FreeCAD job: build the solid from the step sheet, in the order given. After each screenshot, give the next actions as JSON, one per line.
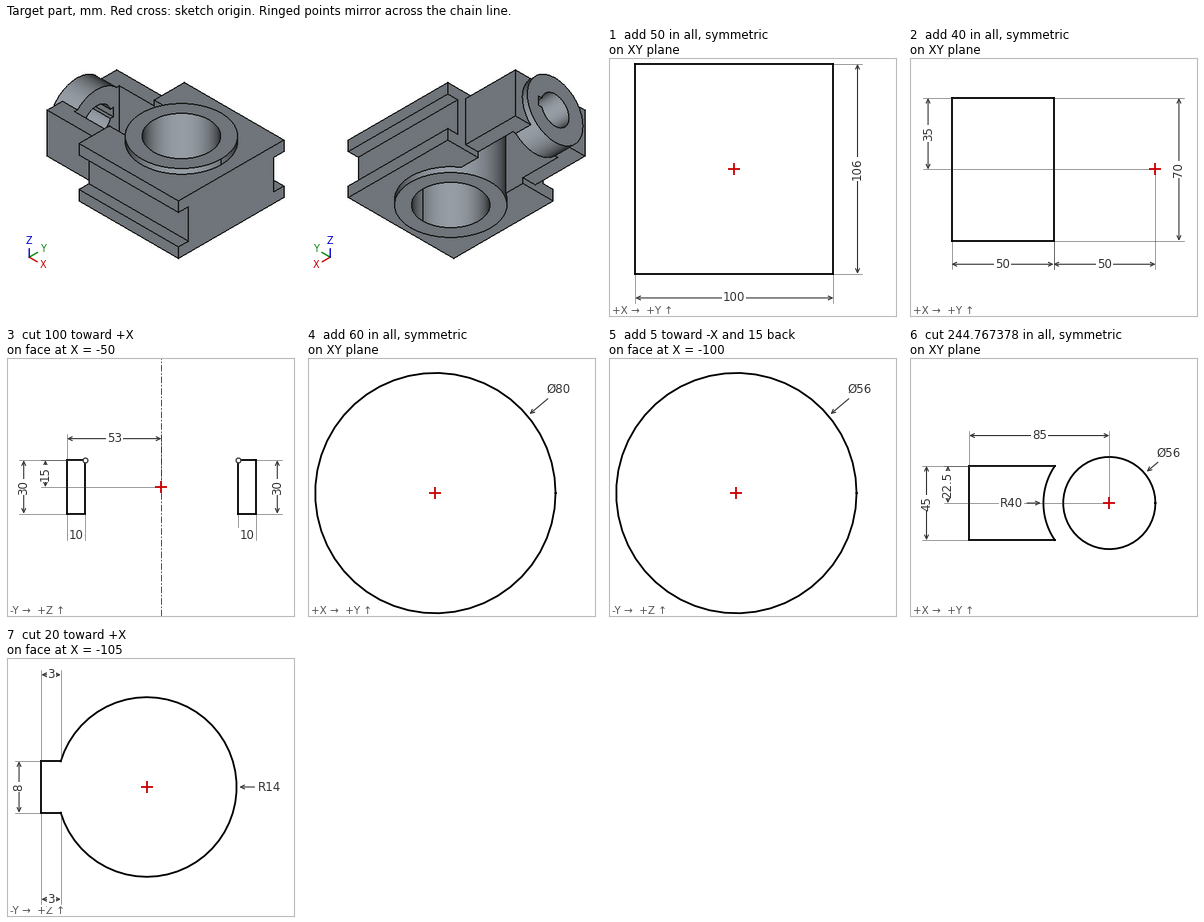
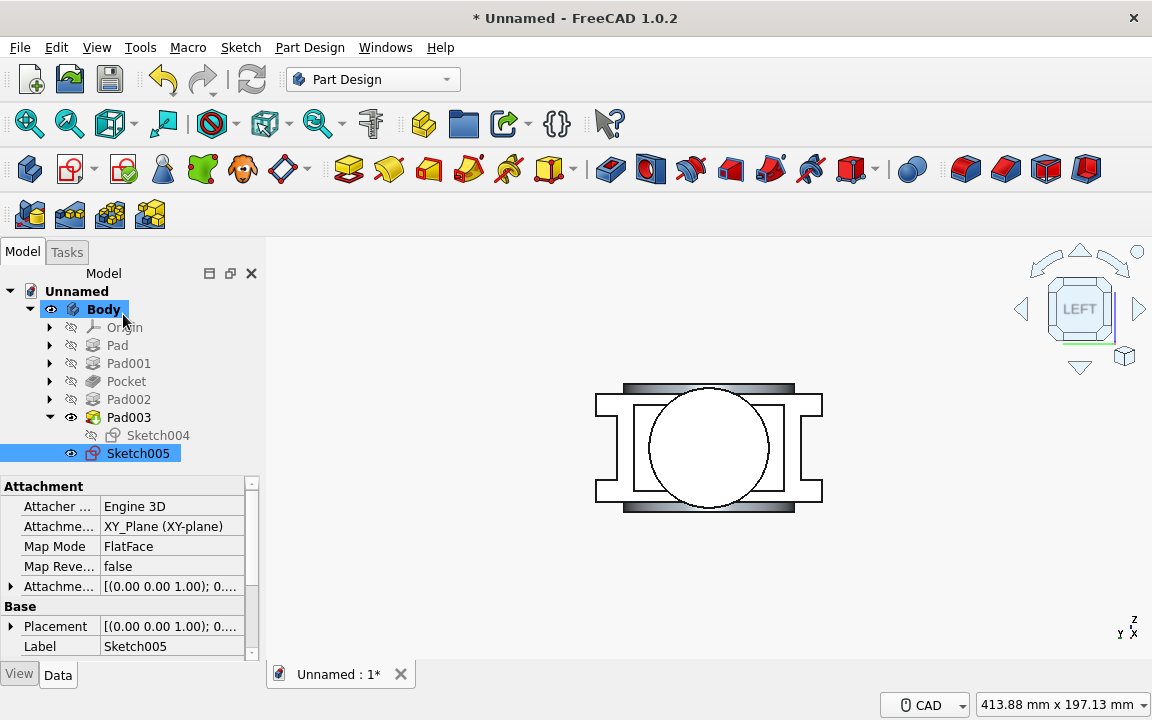
{"action": "left_click", "coordinate": [612, 170]}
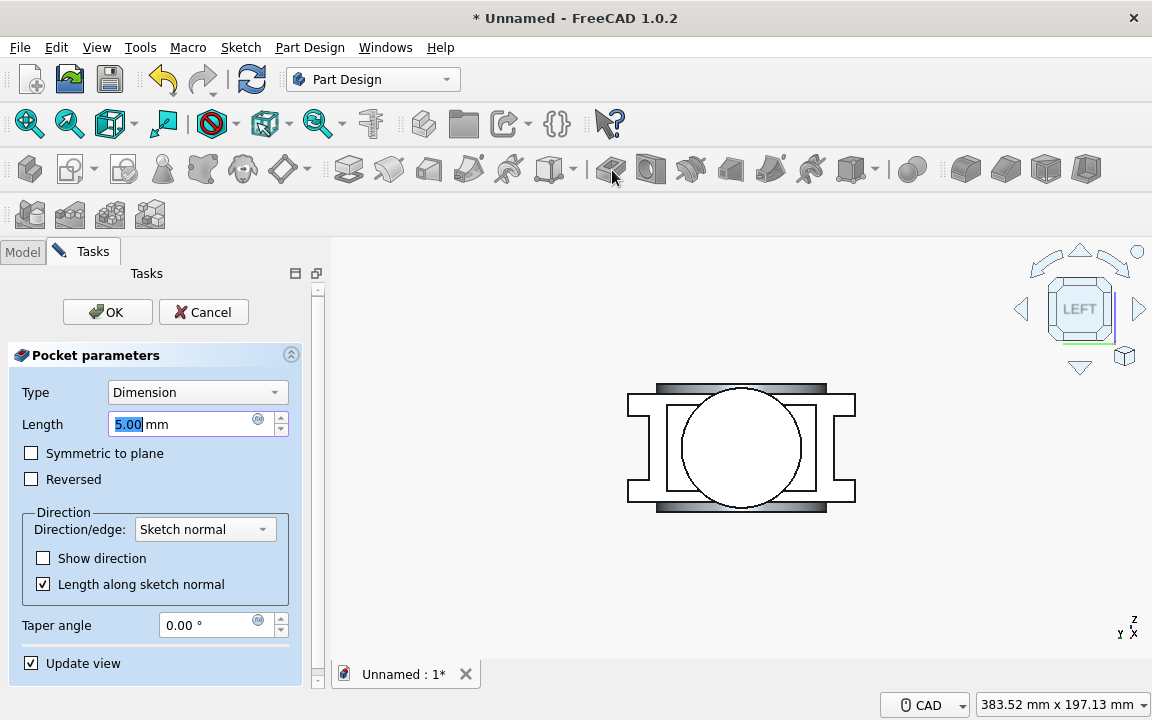
{"action": "type", "text": "244.767378"}
{"action": "key", "text": "Tab"}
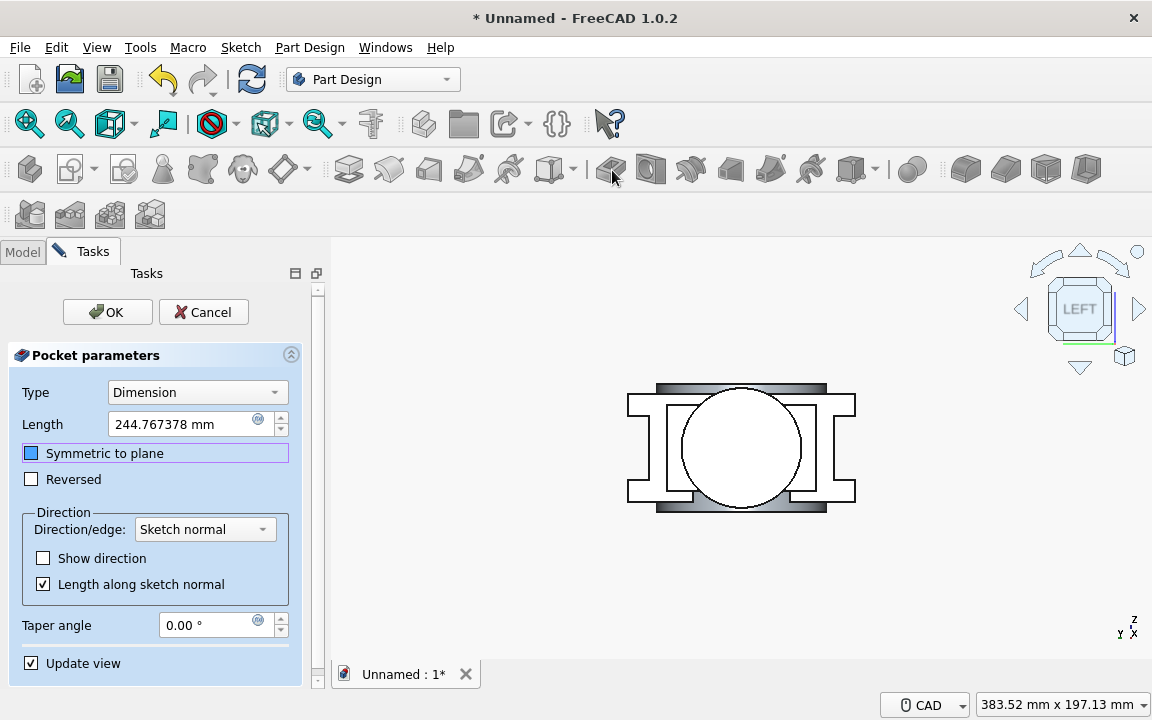
{"action": "left_click", "coordinate": [30, 453]}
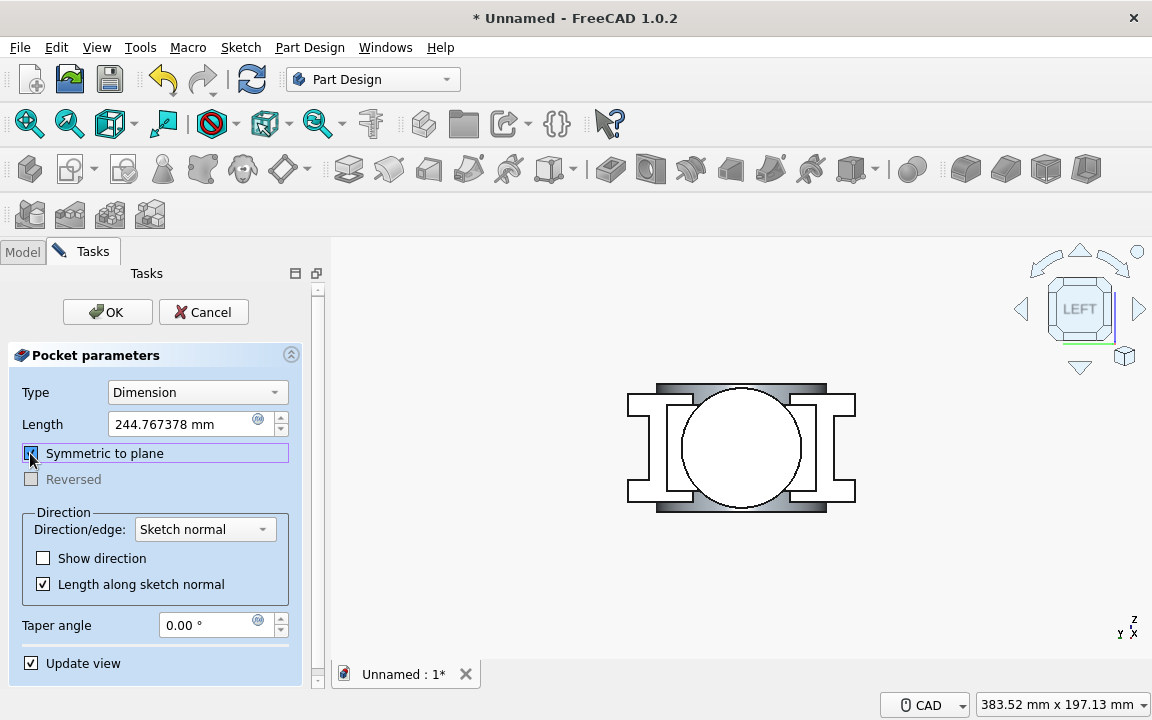
{"action": "left_click", "coordinate": [108, 312]}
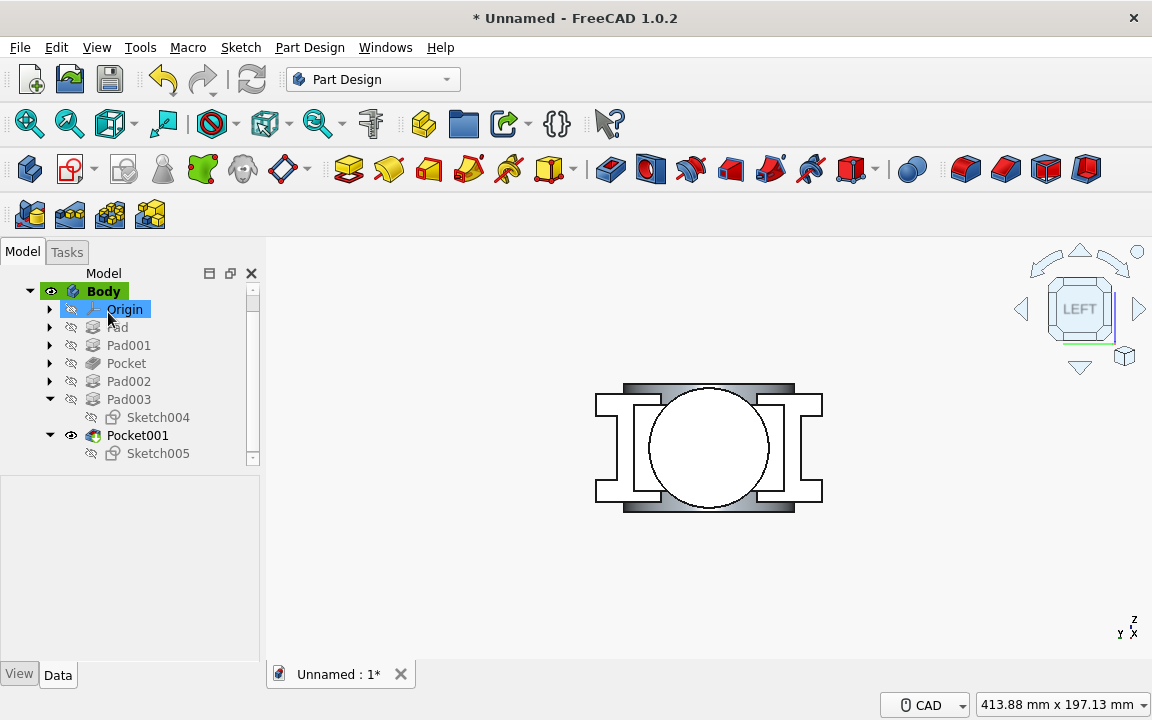
{"action": "left_click", "coordinate": [30, 124]}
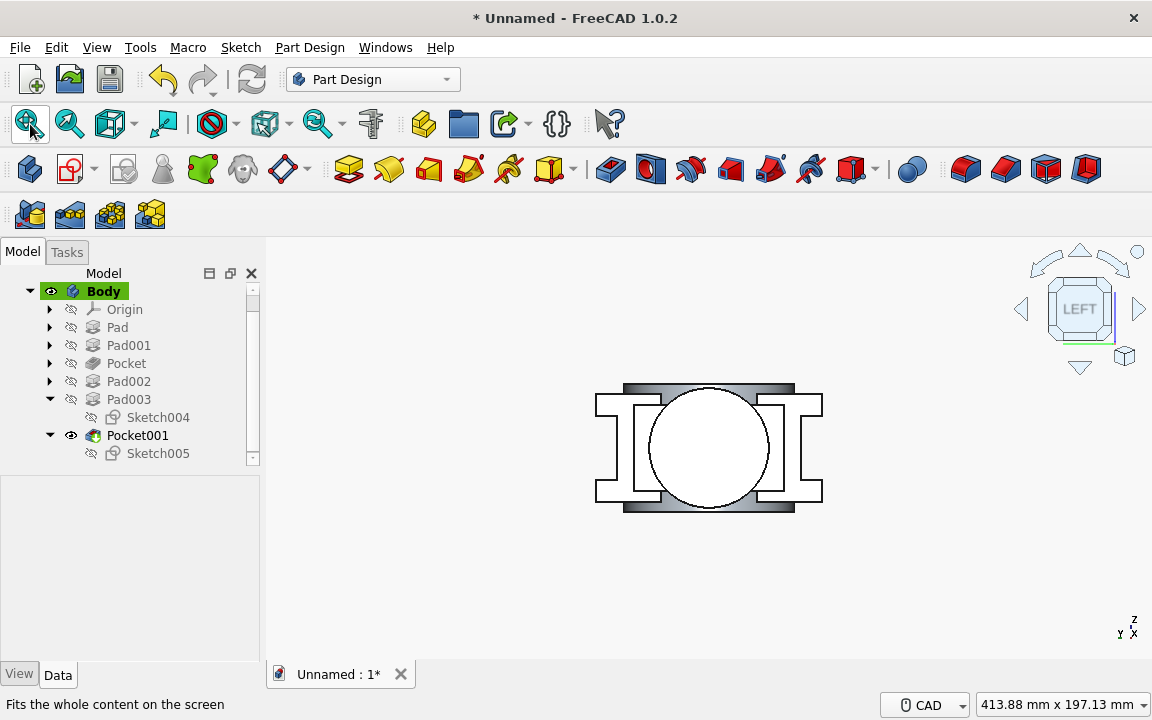
{"action": "left_click", "coordinate": [709, 447]}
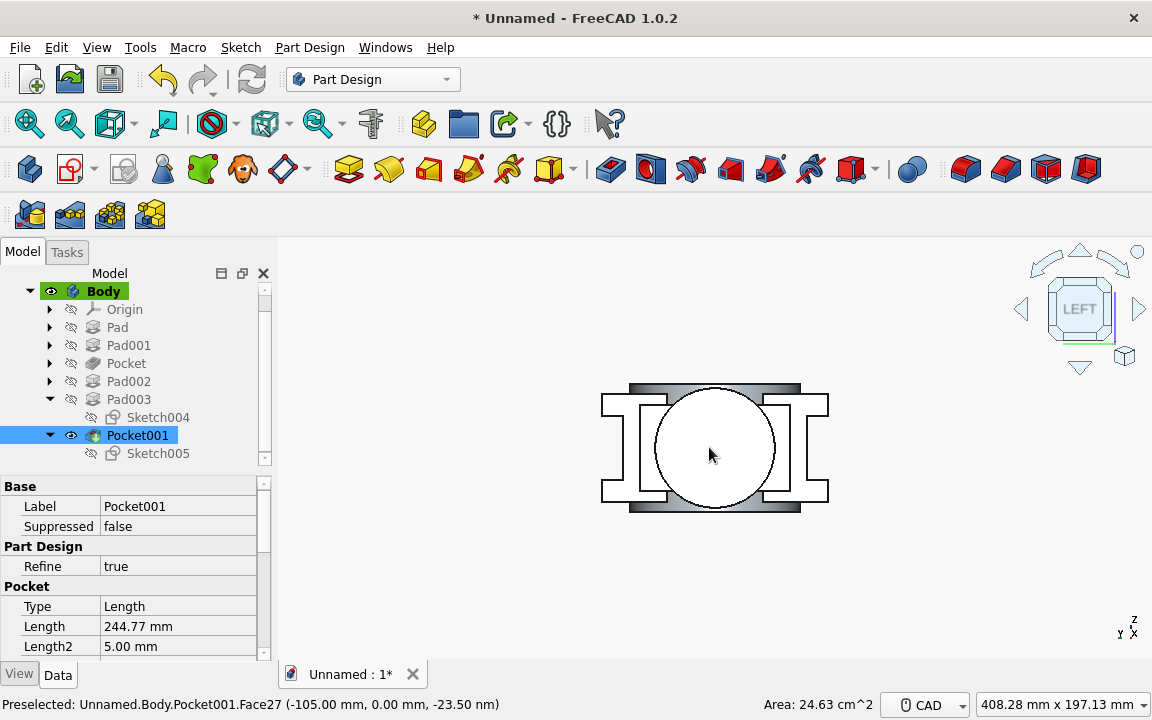
{"action": "left_click", "coordinate": [70, 170]}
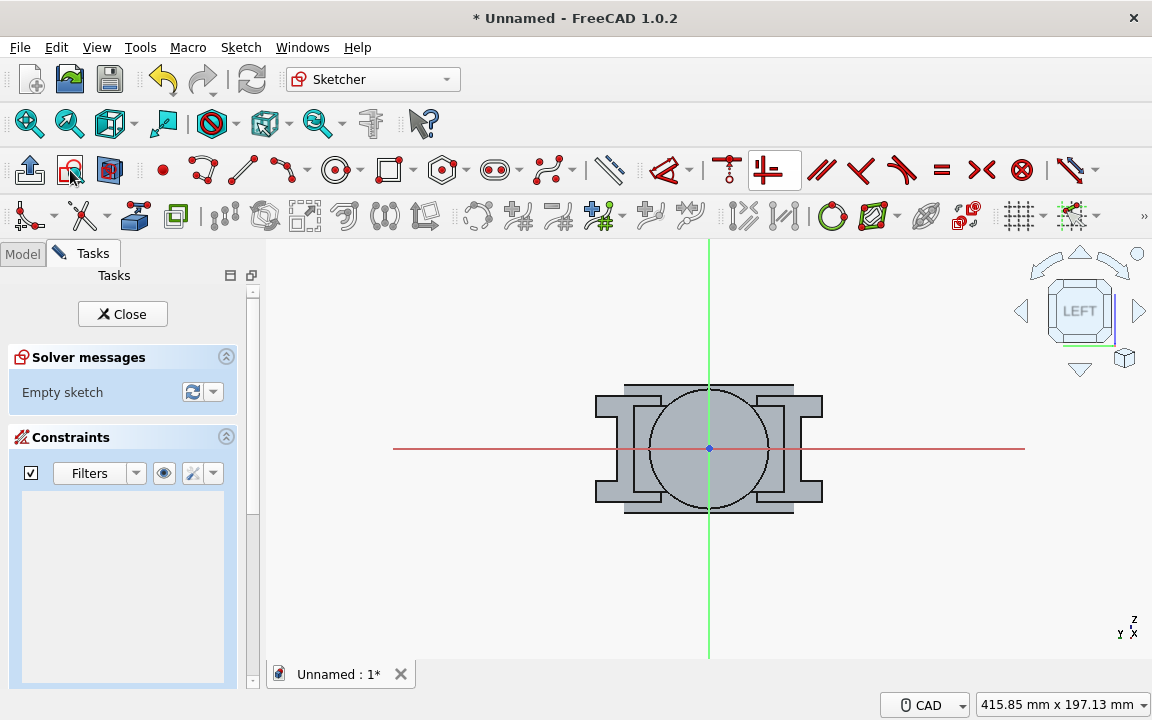
{"action": "scroll", "coordinate": [717, 449], "scroll_direction": "up", "scroll_amount": 10}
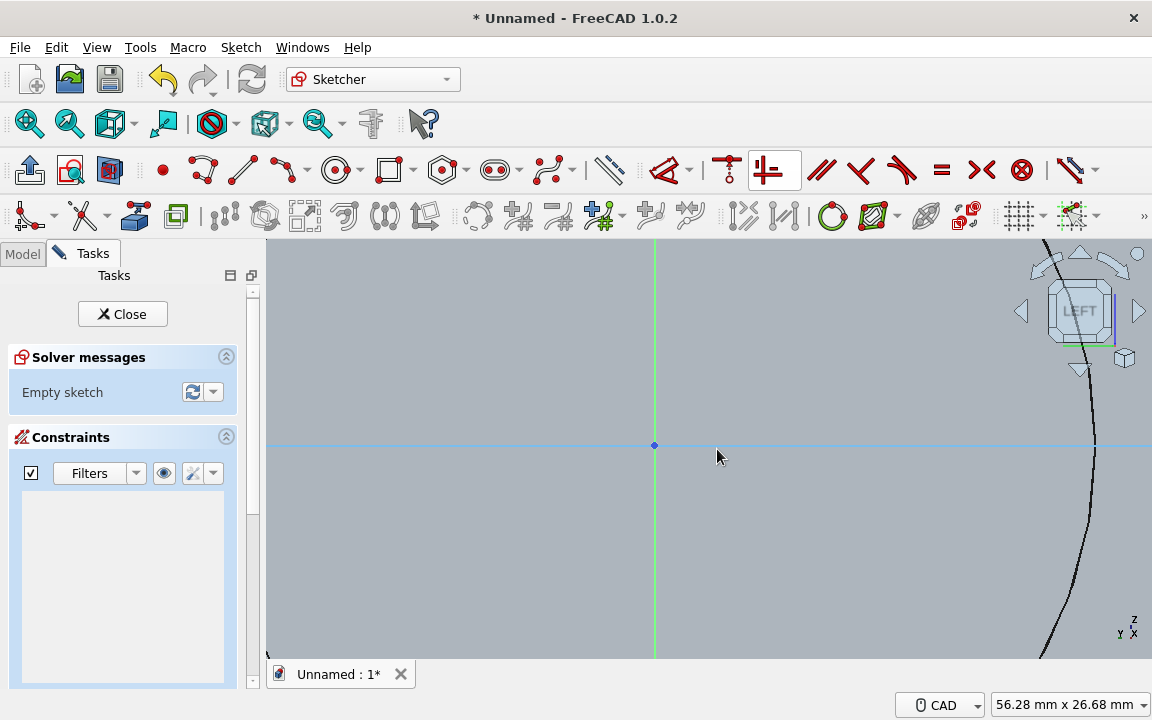
{"action": "left_click", "coordinate": [204, 170]}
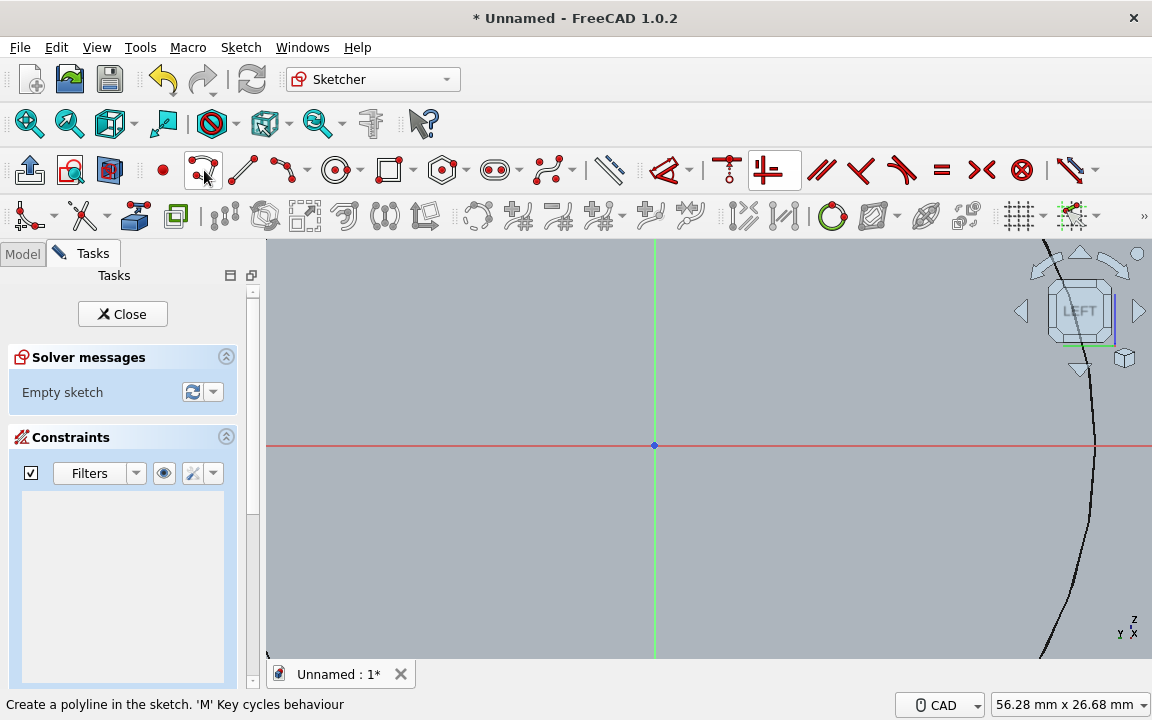
{"action": "left_click", "coordinate": [443, 383]}
{"action": "left_click", "coordinate": [396, 383]}
{"action": "left_click", "coordinate": [396, 509]}
{"action": "left_click", "coordinate": [443, 509]}
{"action": "right_click", "coordinate": [443, 509]}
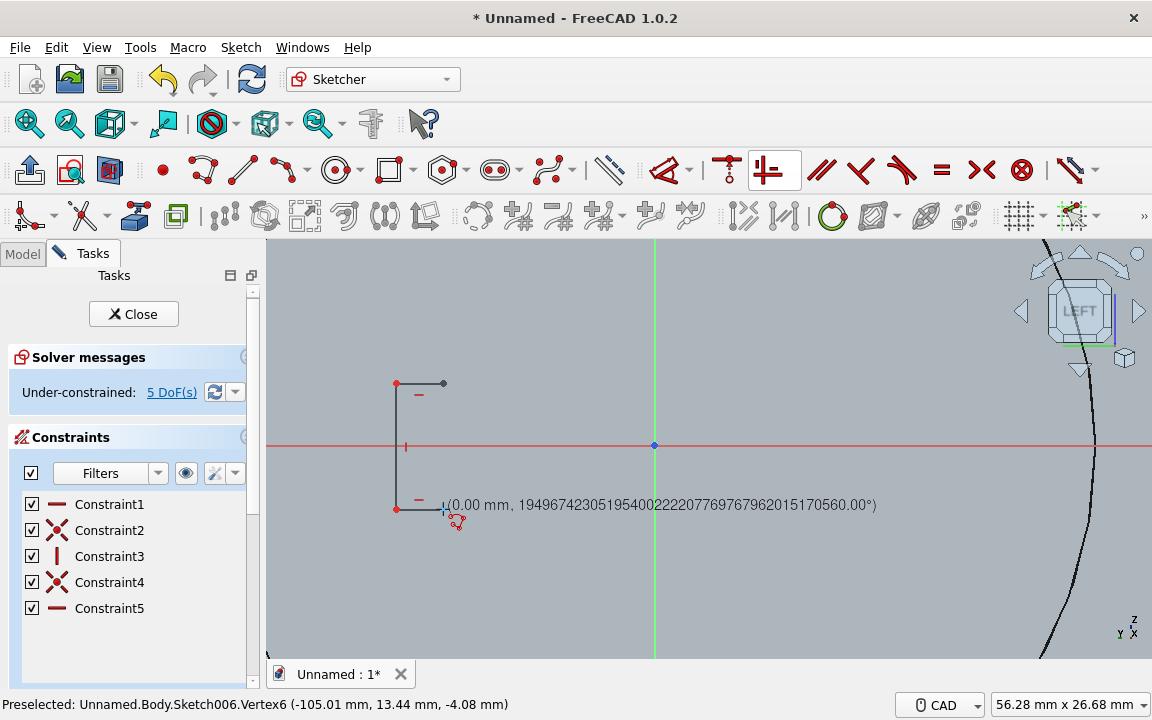
{"action": "left_click", "coordinate": [284, 170]}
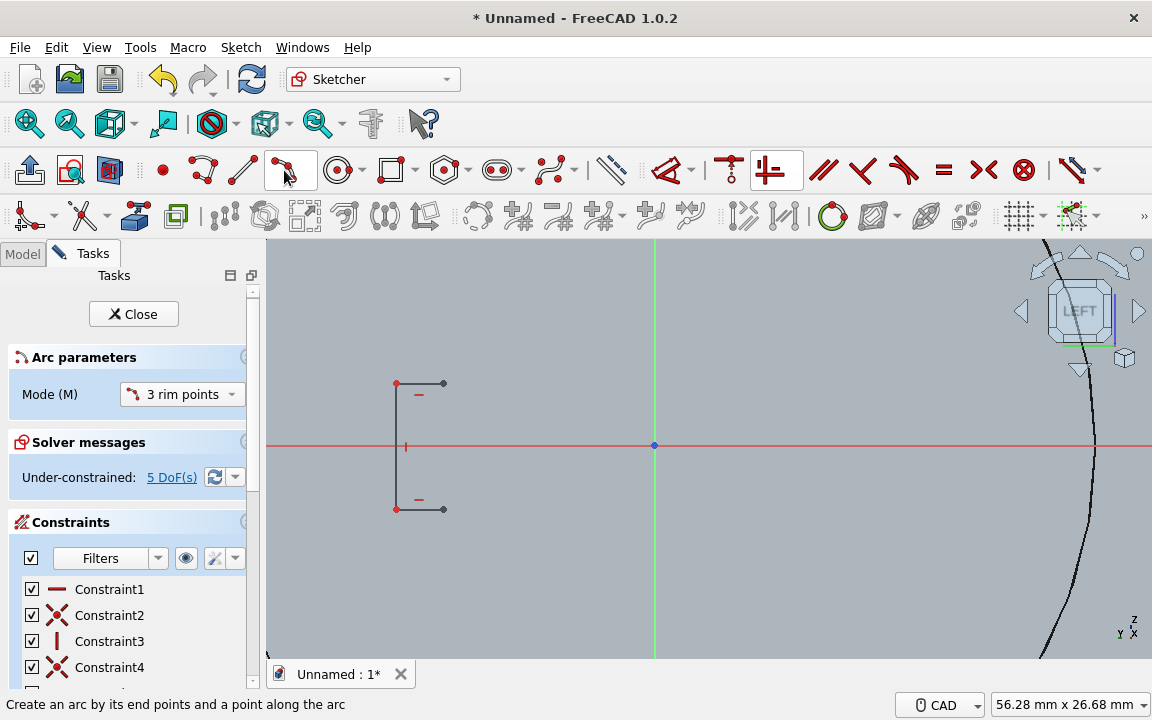
{"action": "left_click", "coordinate": [443, 510]}
{"action": "left_click", "coordinate": [443, 384]}
{"action": "left_click", "coordinate": [840, 565]}
{"action": "key", "text": "Escape"}